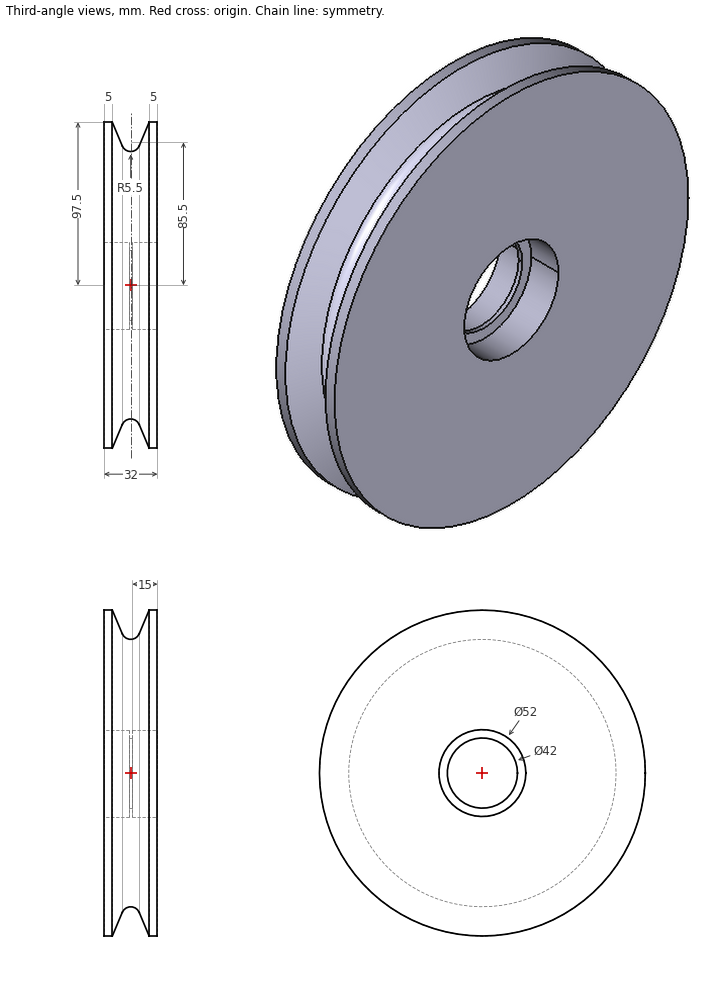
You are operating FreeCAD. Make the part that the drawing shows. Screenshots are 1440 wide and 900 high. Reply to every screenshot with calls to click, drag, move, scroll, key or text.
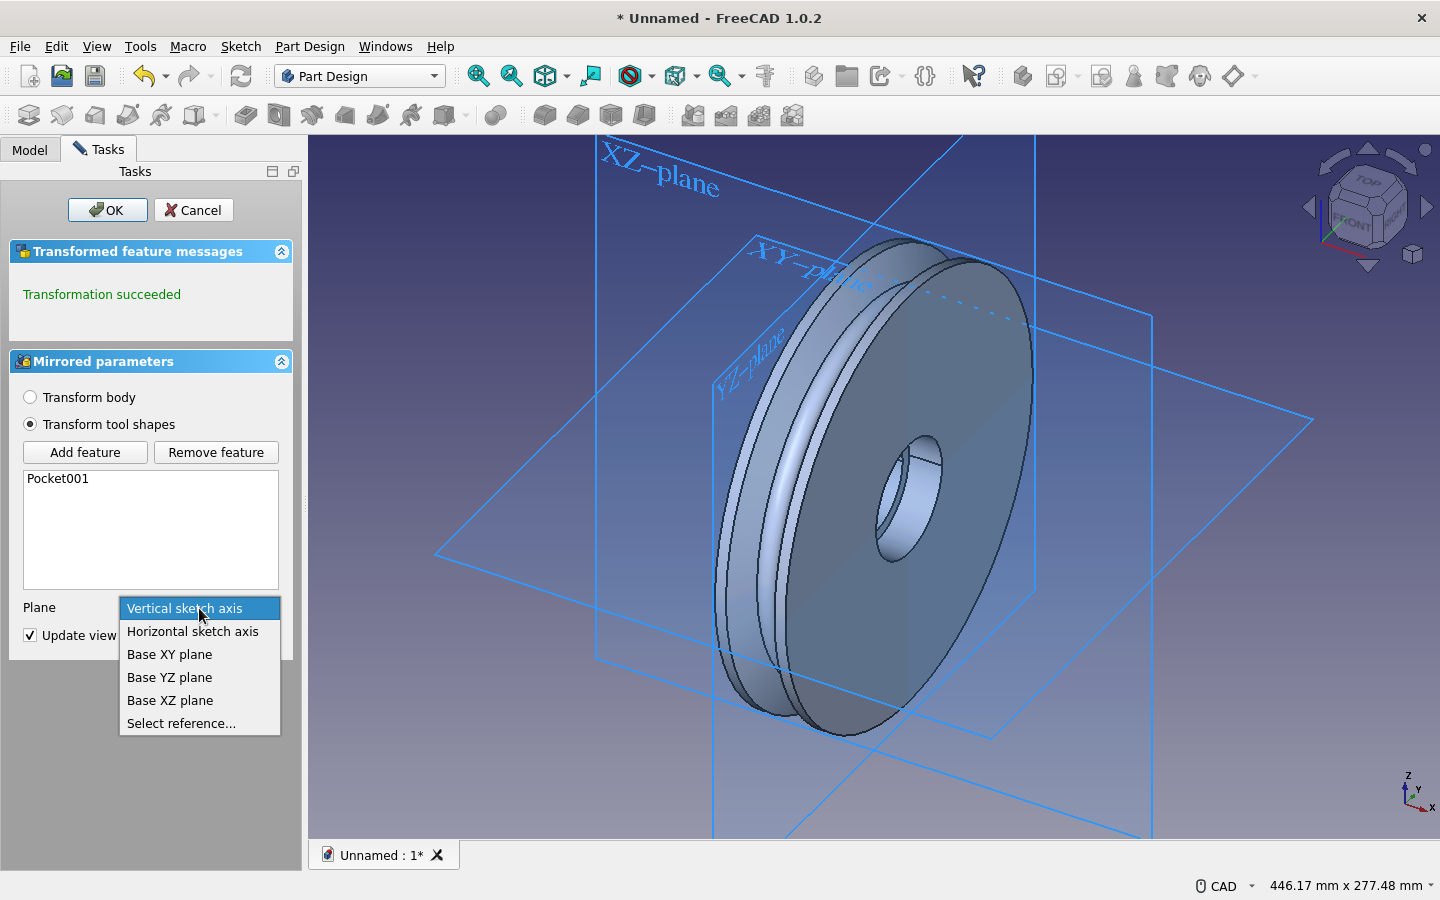
click(198, 678)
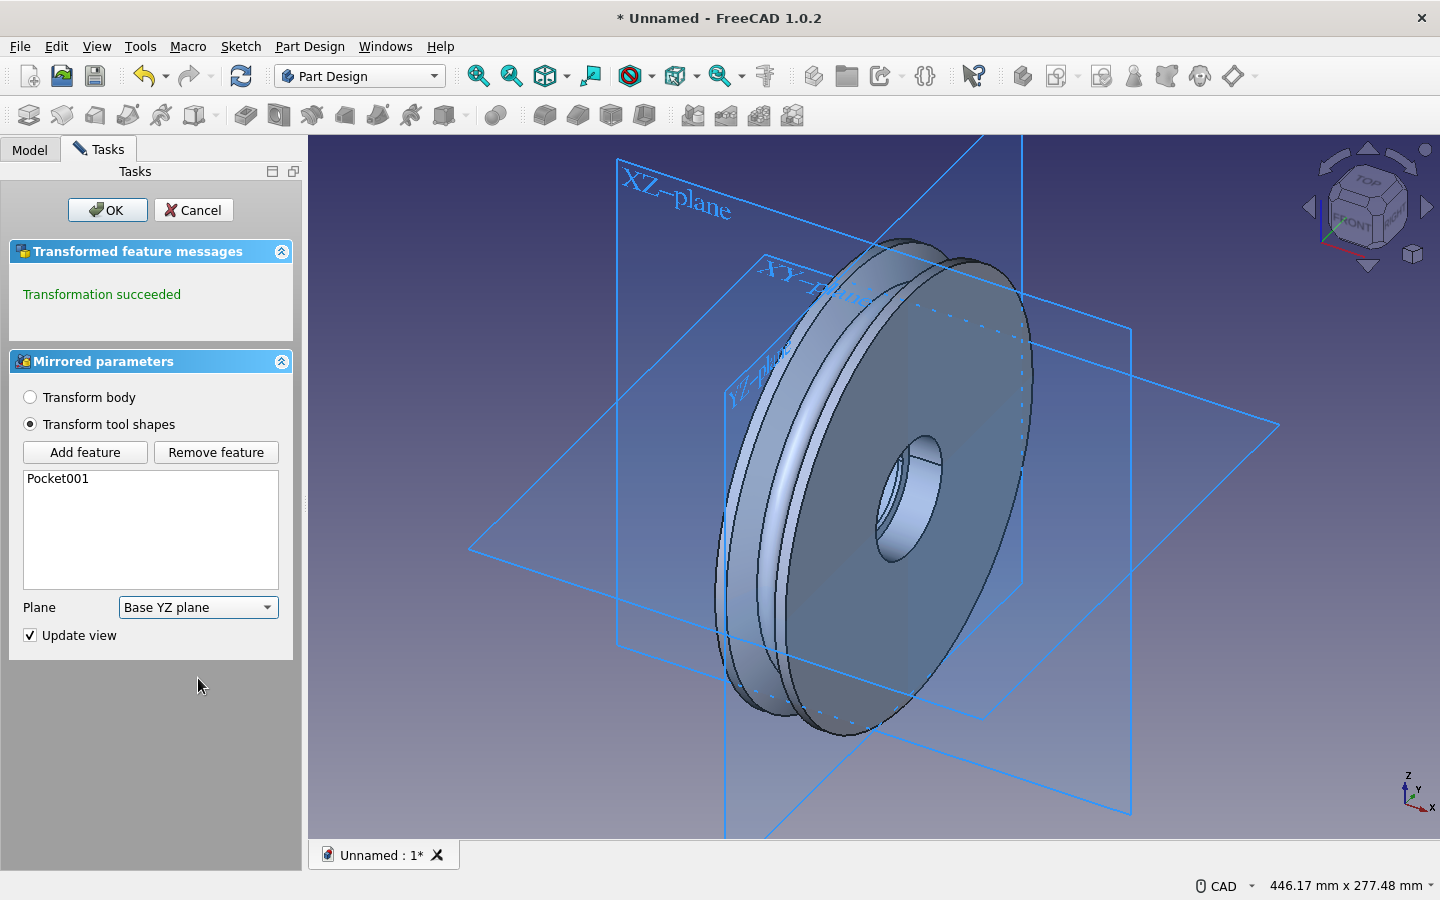
click(108, 210)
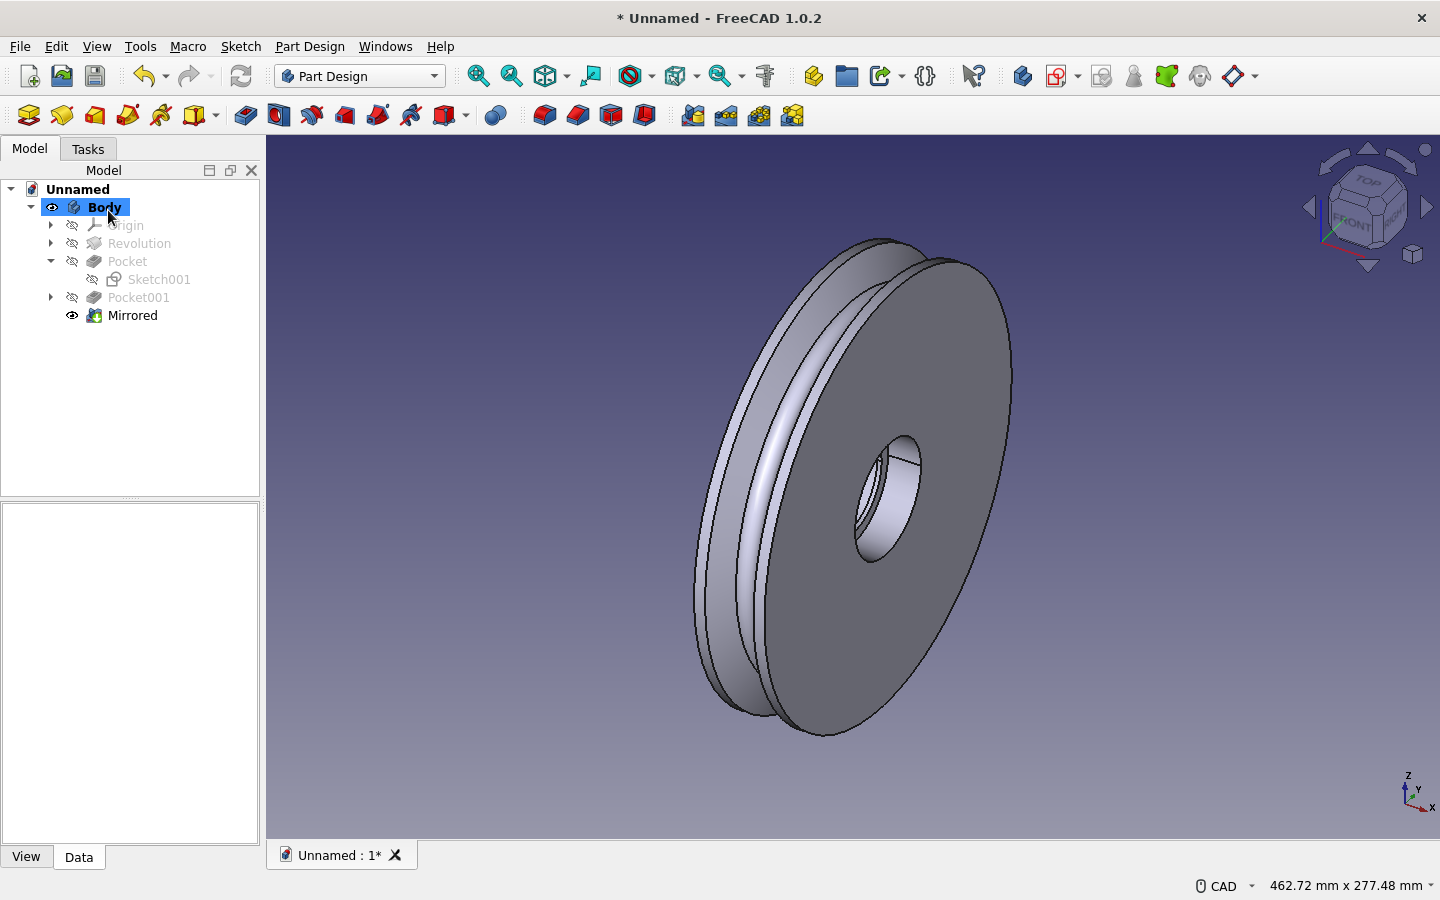
key(0)